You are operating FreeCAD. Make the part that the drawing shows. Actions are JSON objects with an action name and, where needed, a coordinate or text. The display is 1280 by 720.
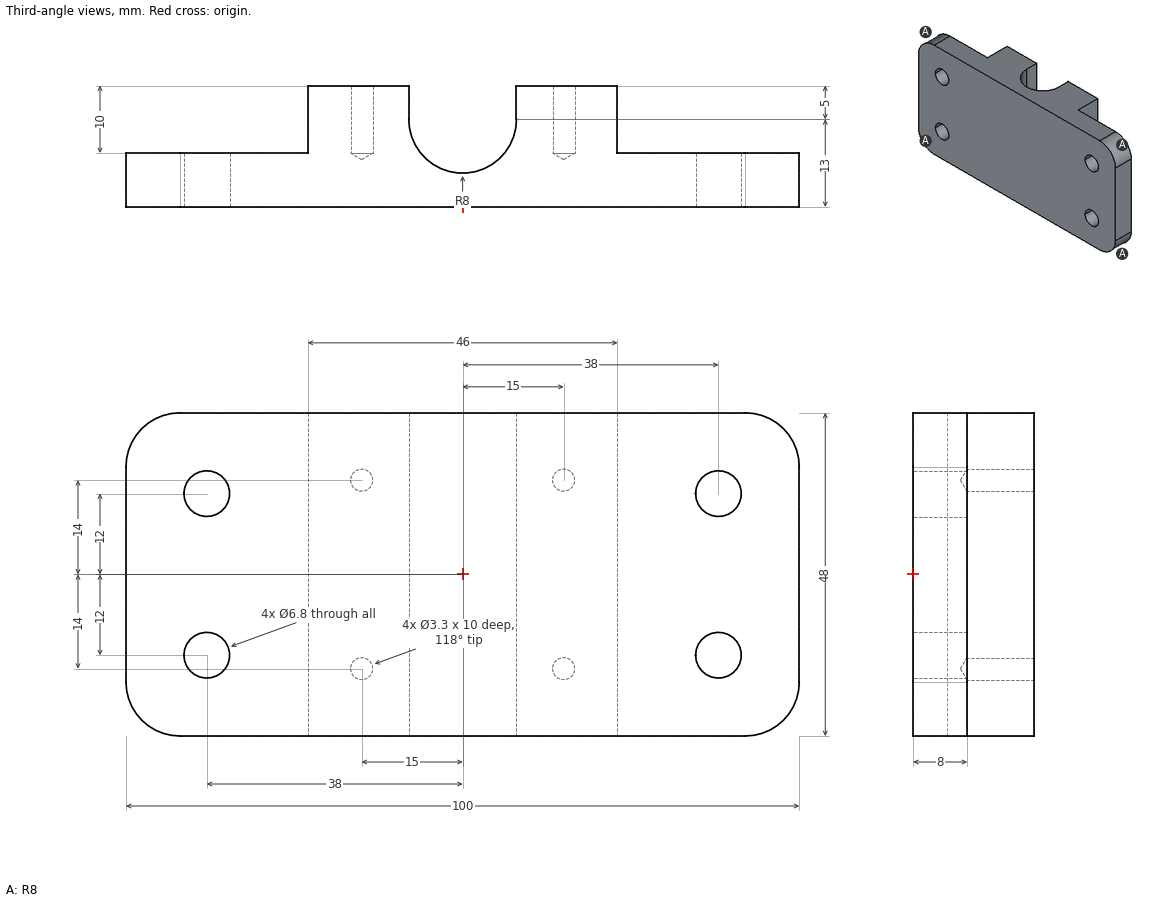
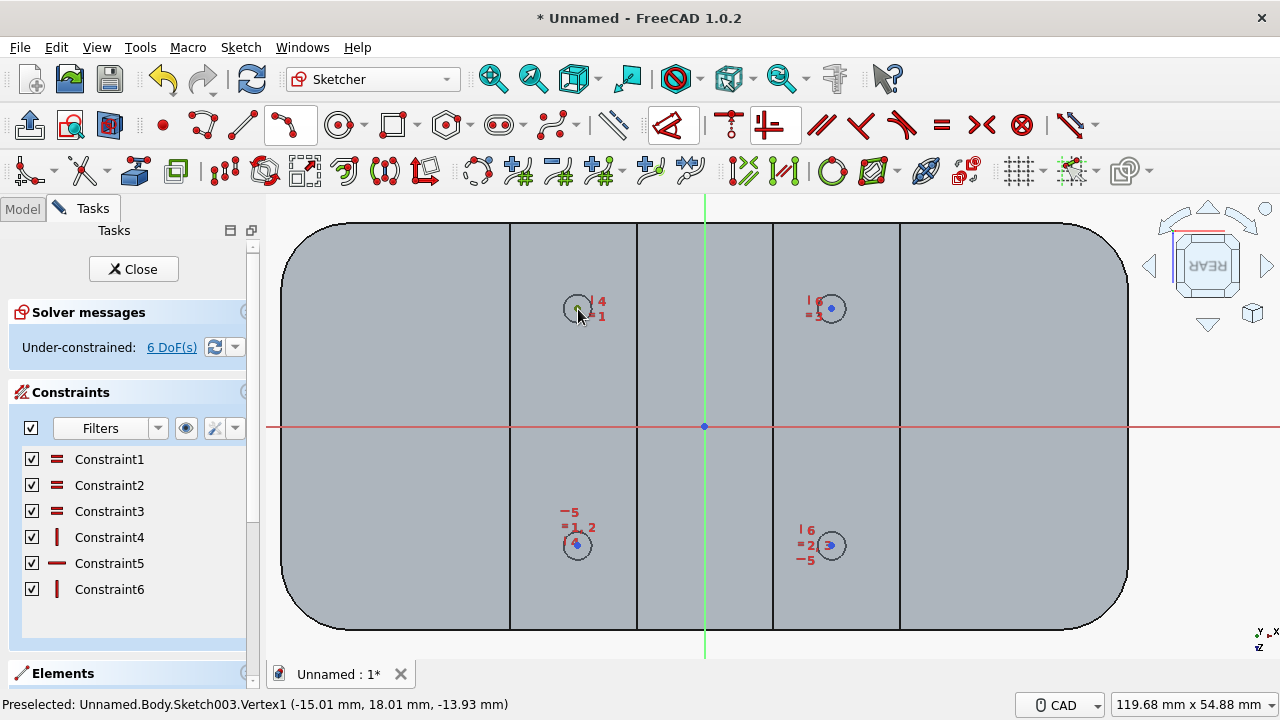
{"action": "left_click", "coordinate": [832, 309]}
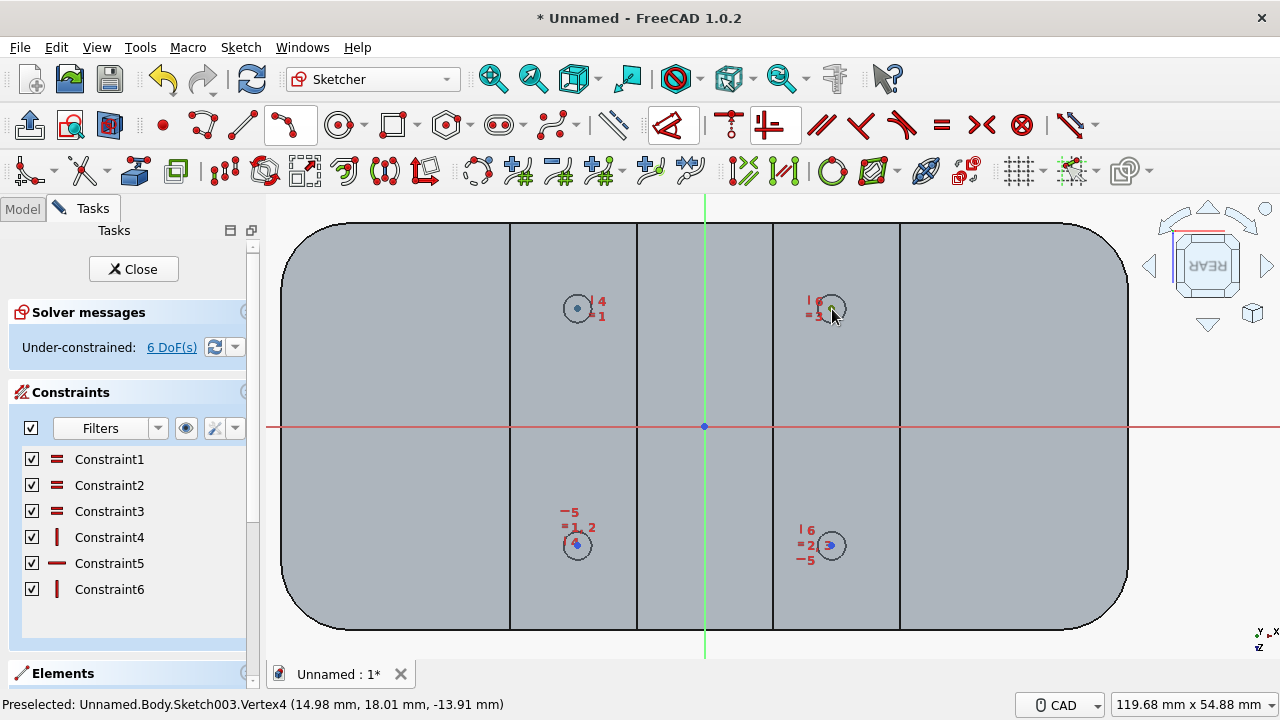
{"action": "key", "text": "h"}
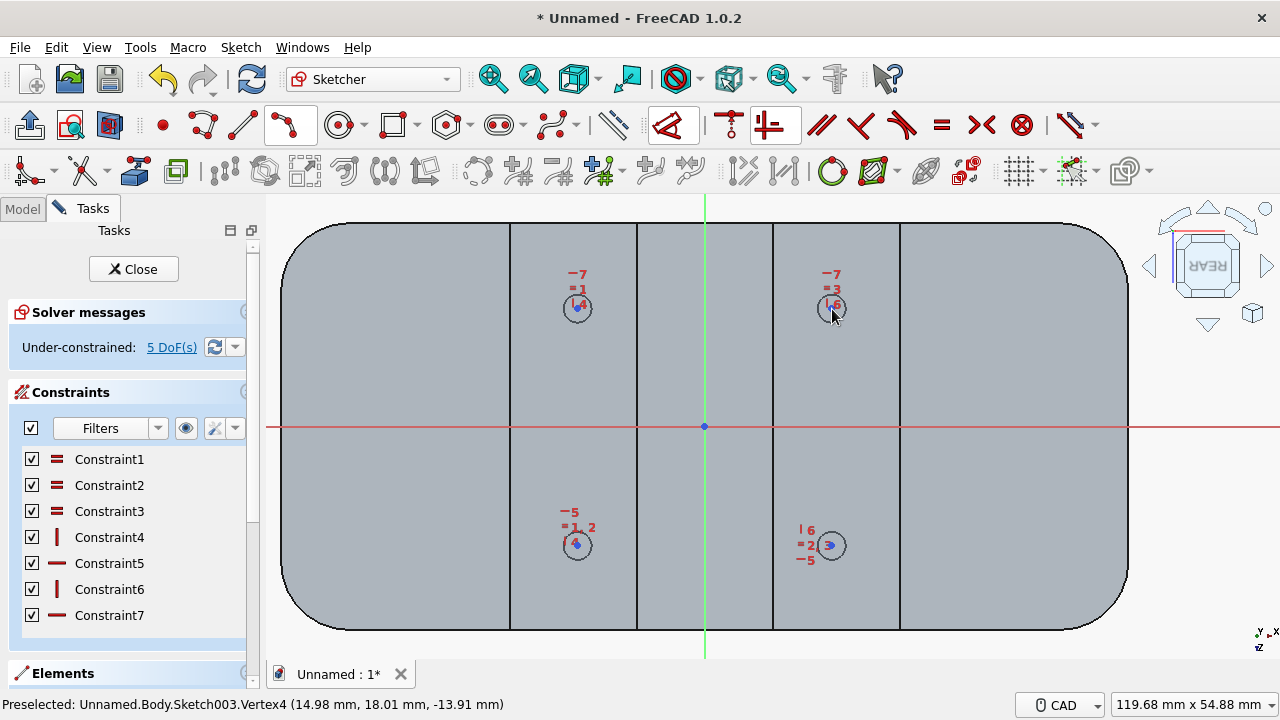
{"action": "scroll", "coordinate": [587, 299], "scroll_direction": "up", "scroll_amount": 2}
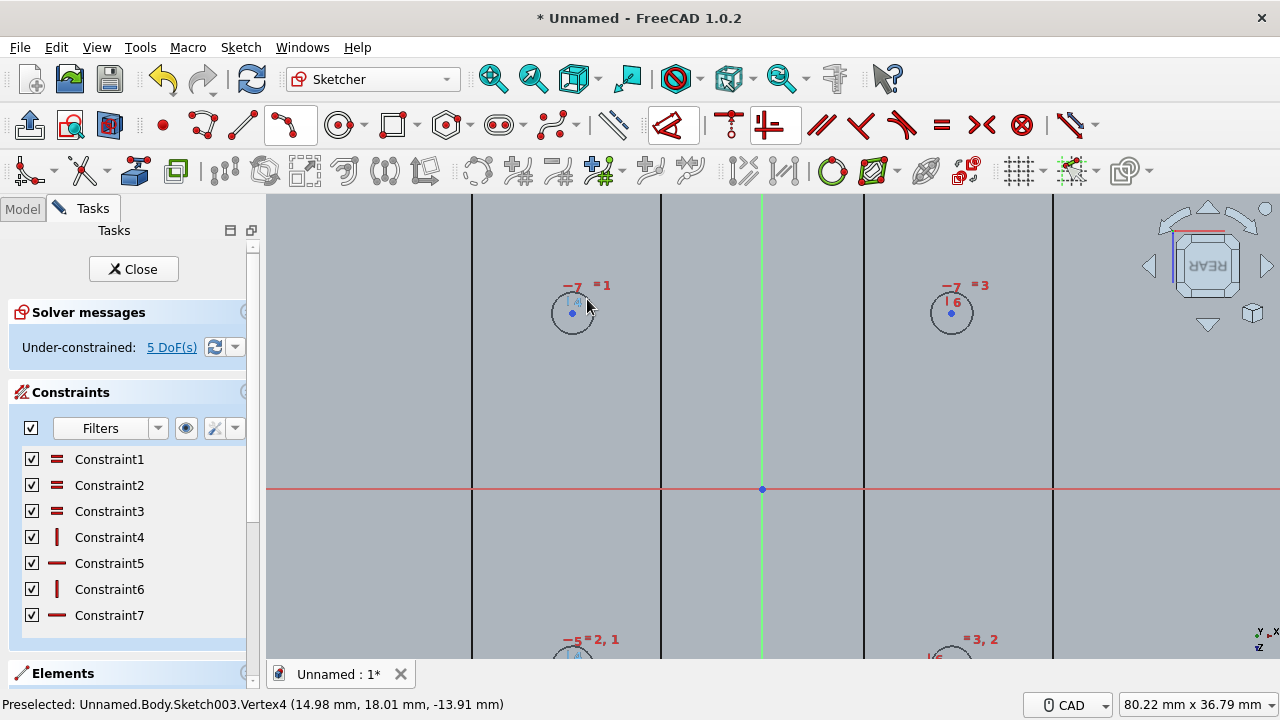
{"action": "left_click", "coordinate": [587, 298]}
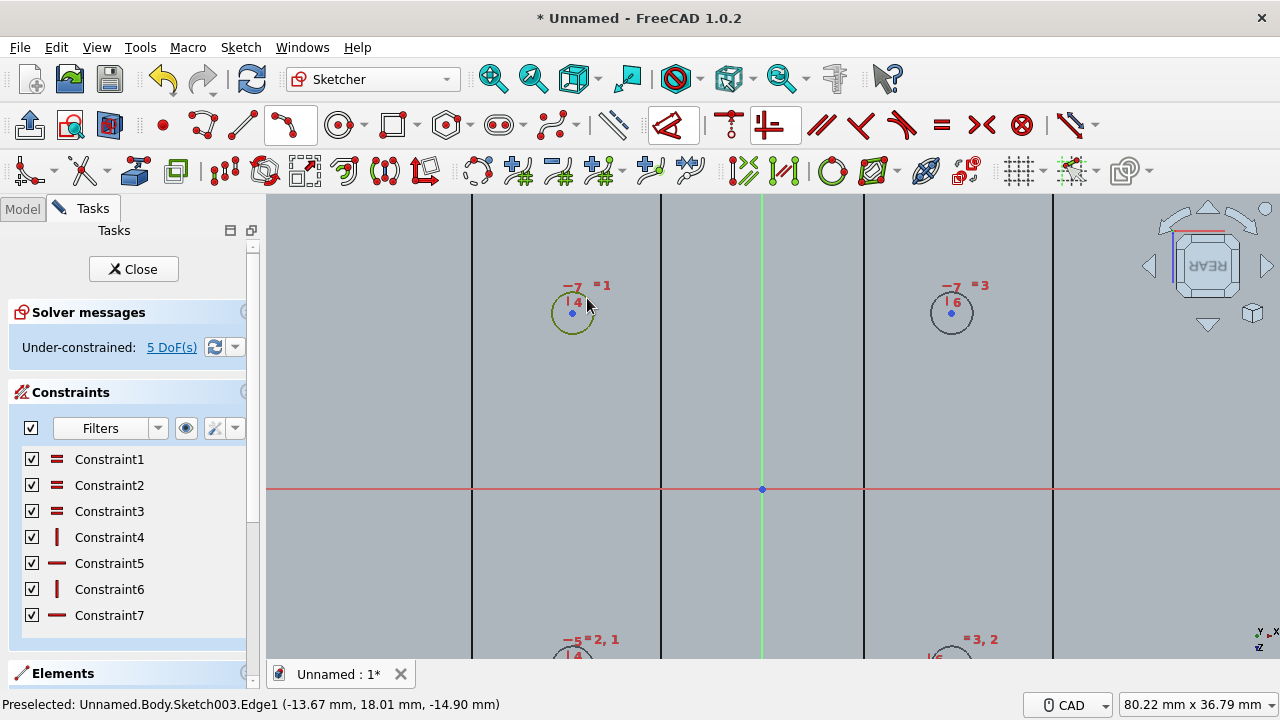
{"action": "left_click", "coordinate": [694, 126]}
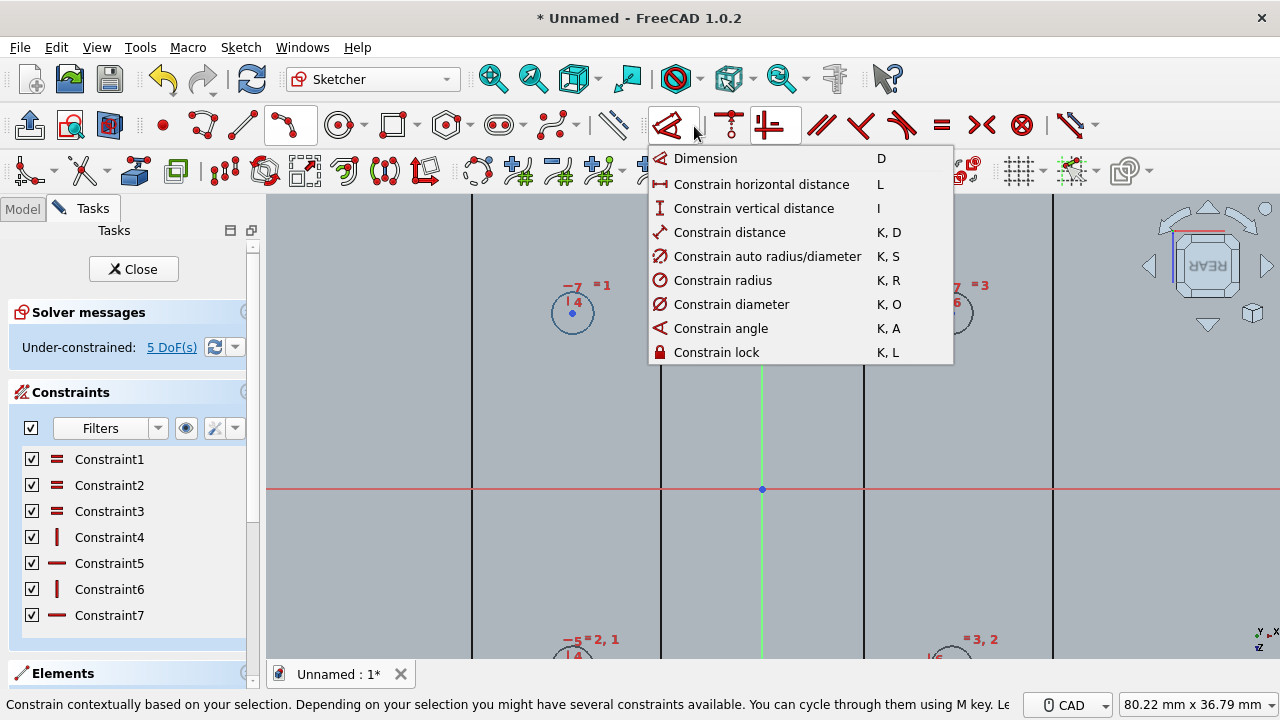
{"action": "left_click", "coordinate": [801, 304]}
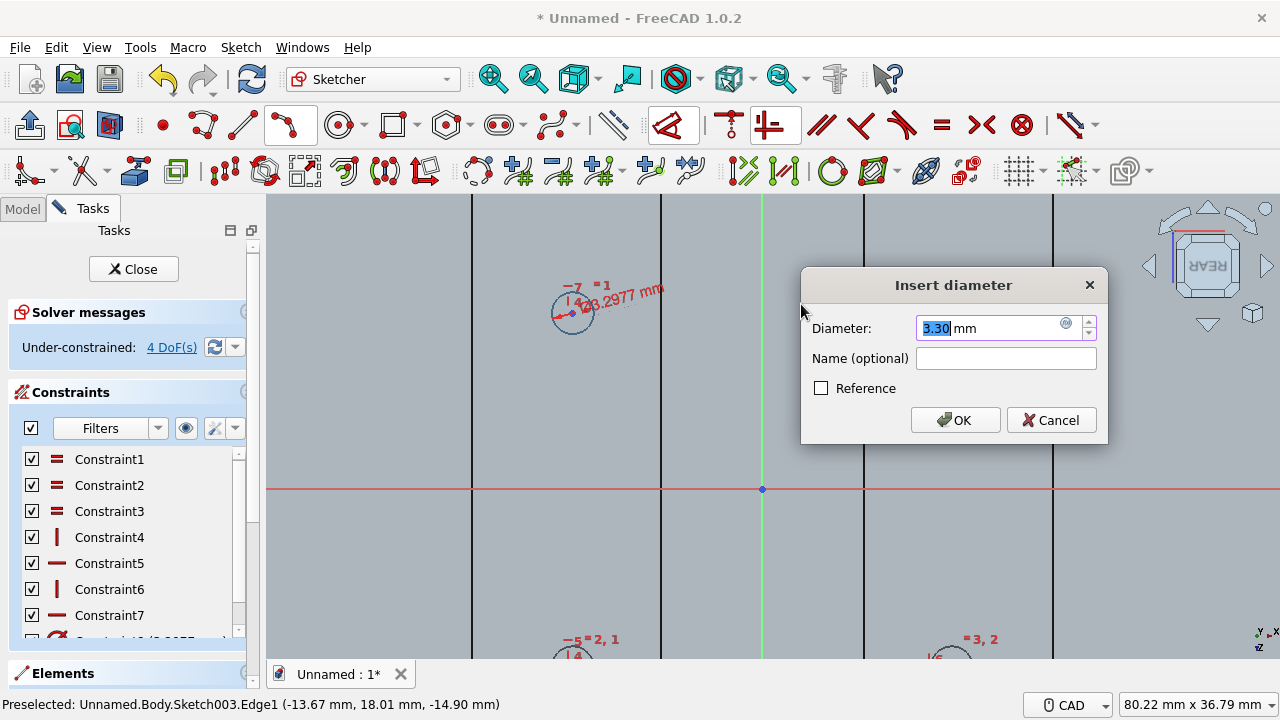
{"action": "type", "text": "3.3"}
{"action": "key", "text": "Return"}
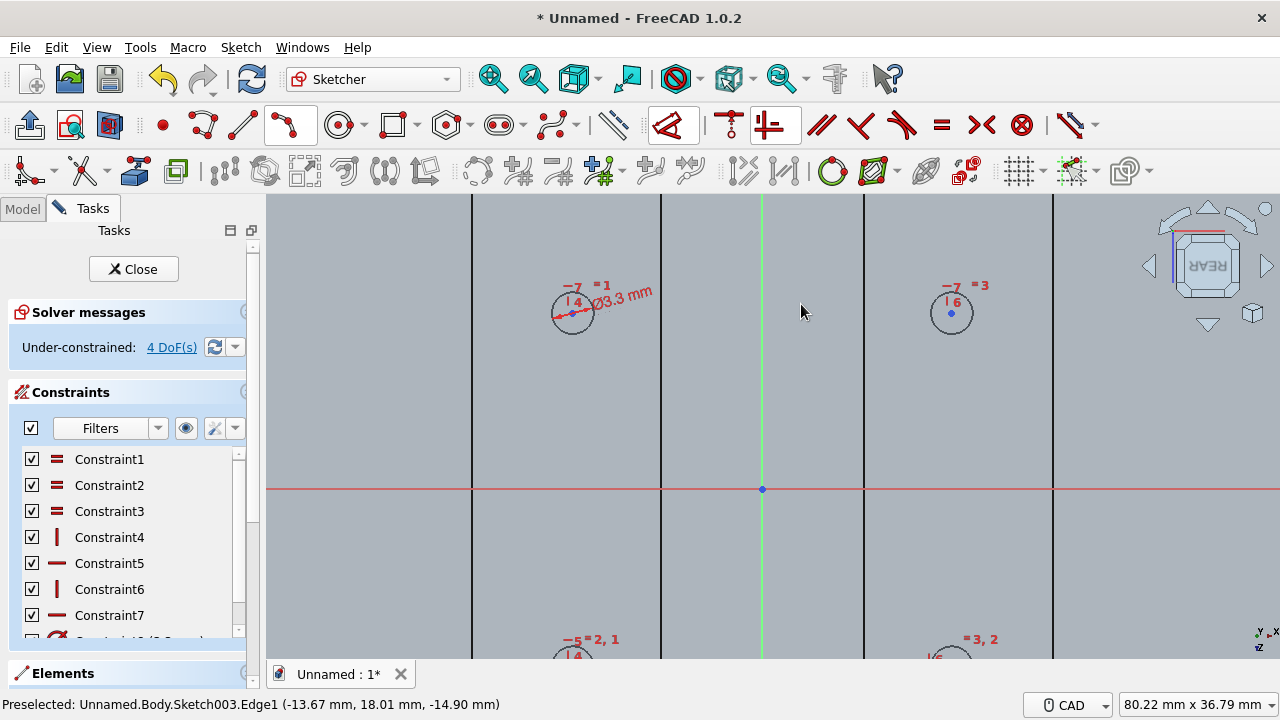
{"action": "left_click", "coordinate": [573, 313]}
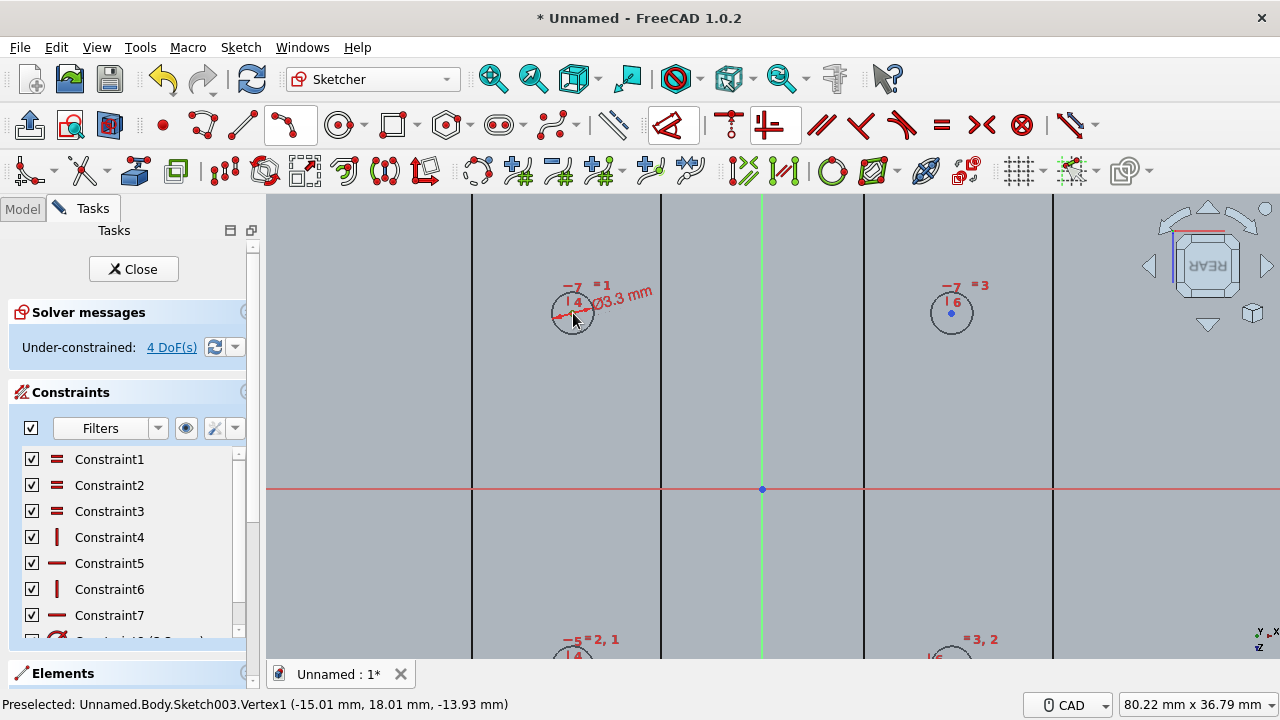
{"action": "left_click", "coordinate": [694, 126]}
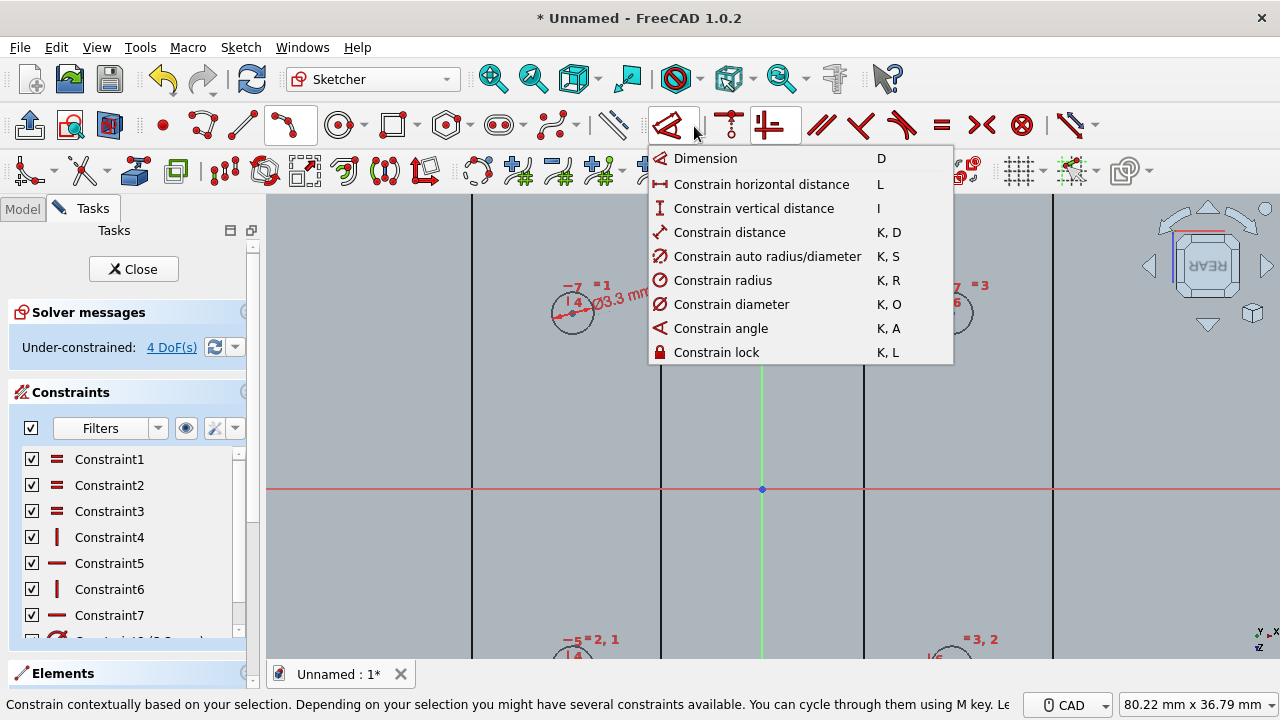
{"action": "left_click", "coordinate": [801, 184]}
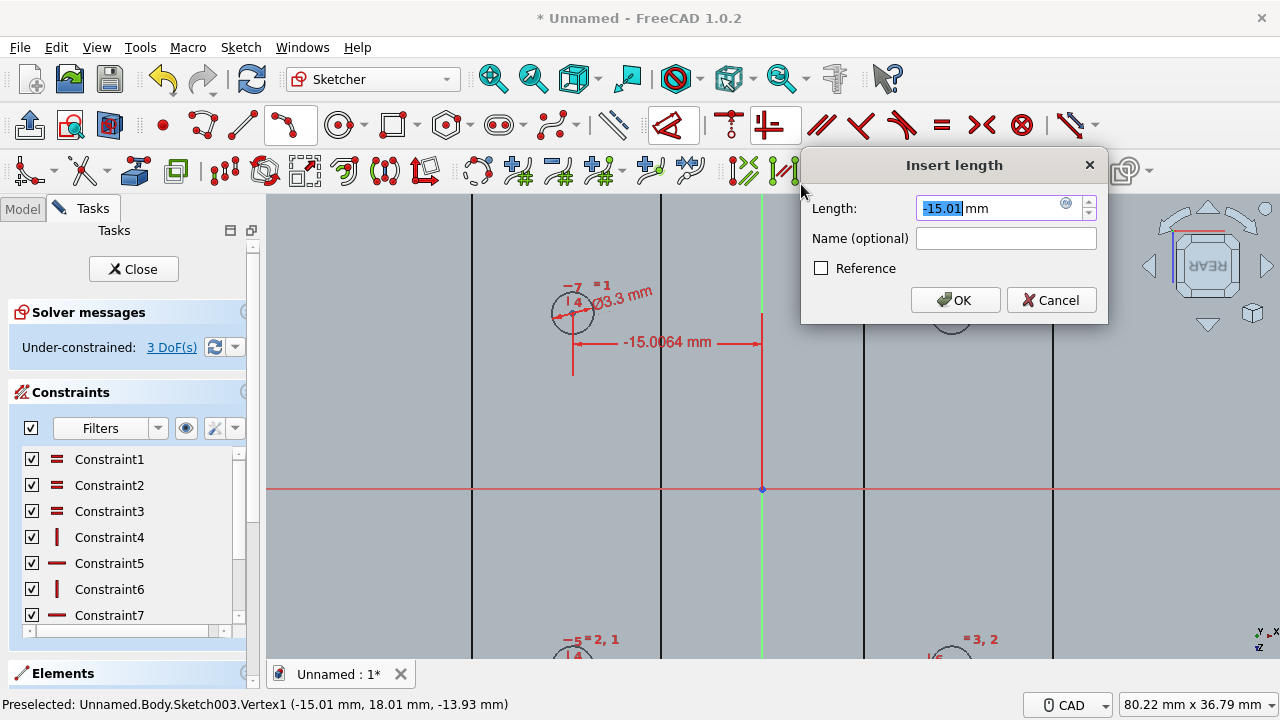
{"action": "type", "text": "-15"}
{"action": "key", "text": "Return"}